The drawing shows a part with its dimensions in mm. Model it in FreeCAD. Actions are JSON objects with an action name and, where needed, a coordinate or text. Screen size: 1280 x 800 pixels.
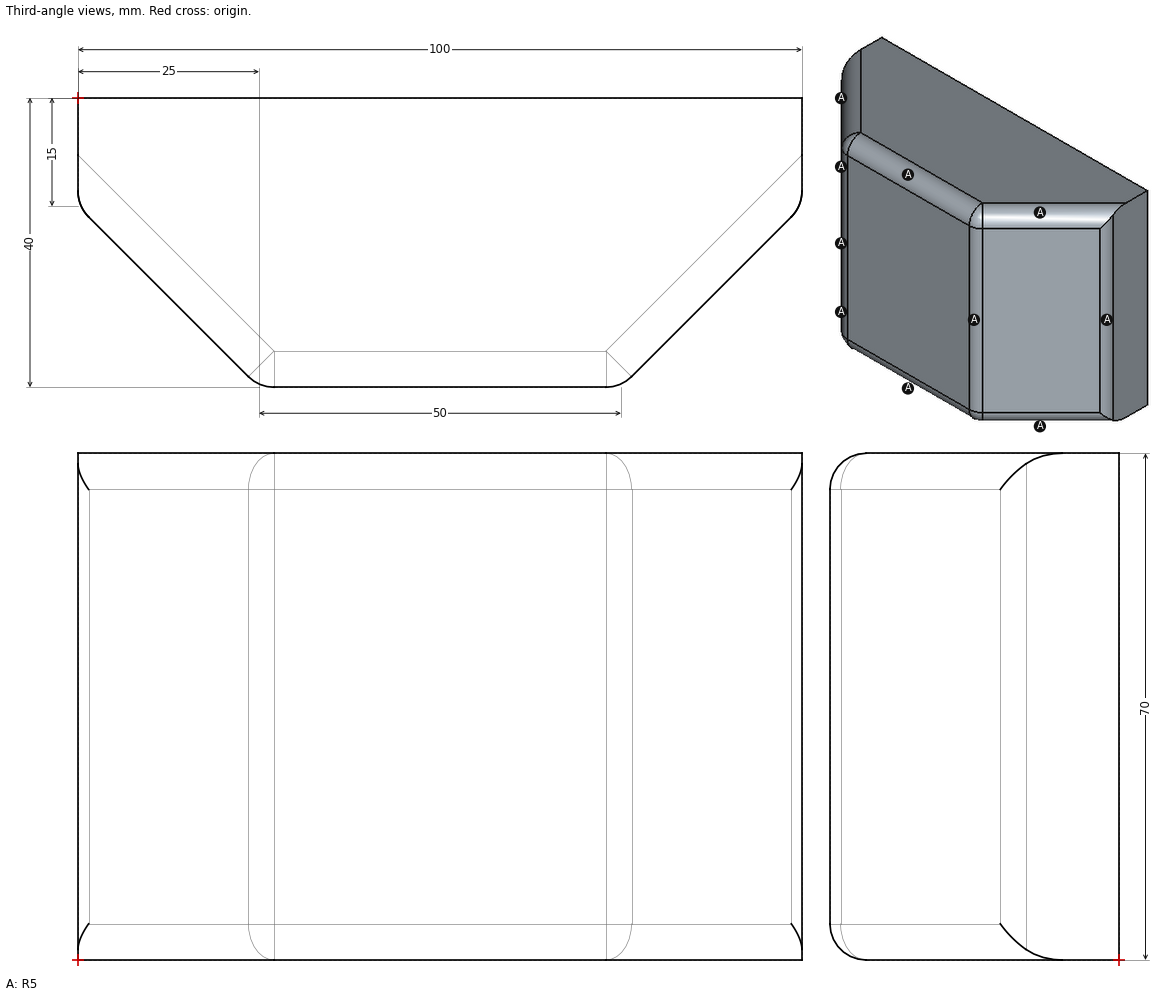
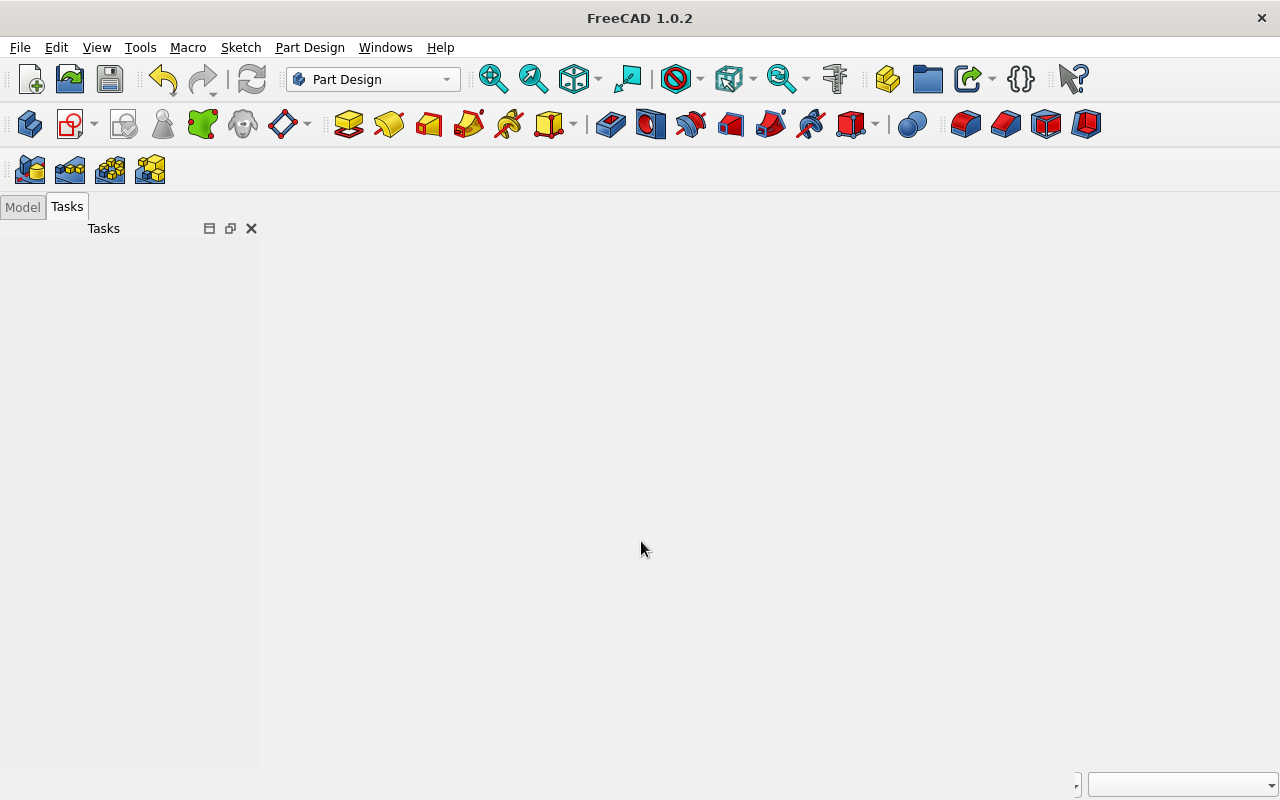
{"action": "key", "text": "ctrl+n"}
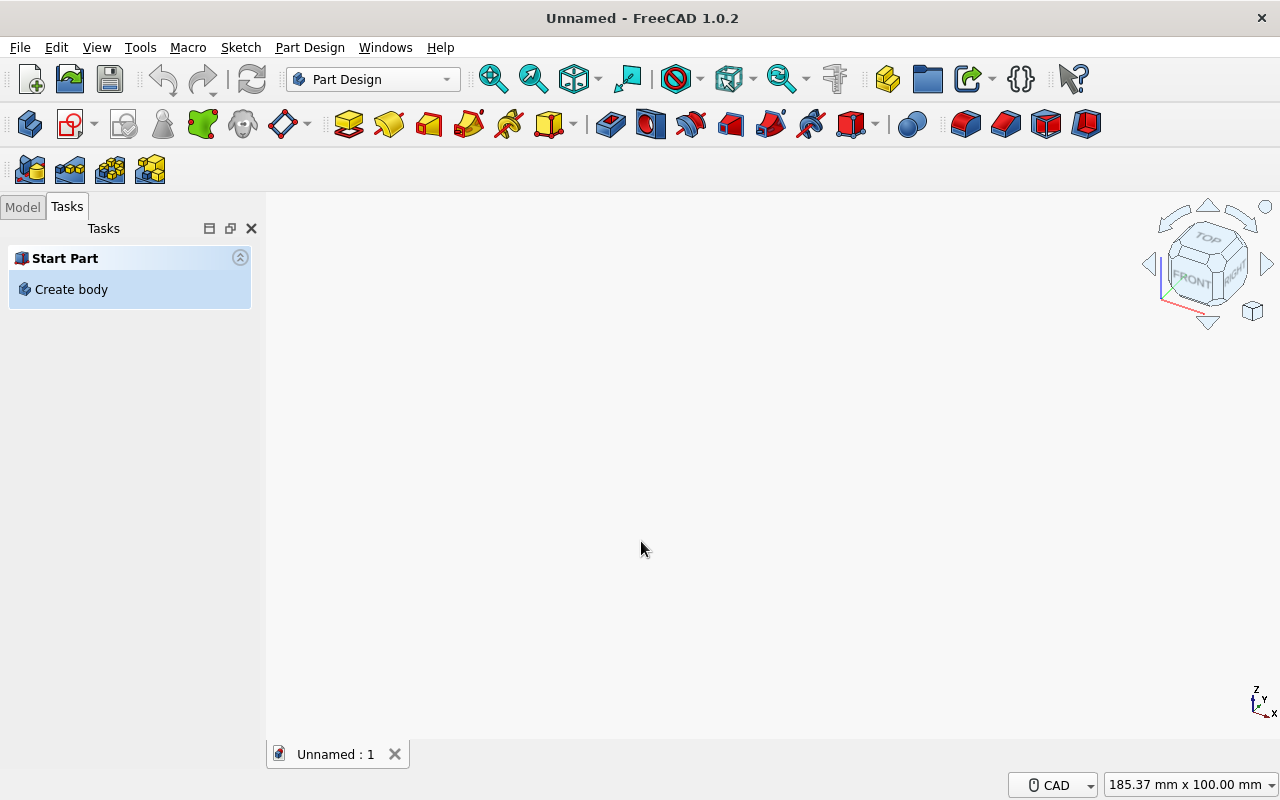
{"action": "left_click", "coordinate": [70, 124]}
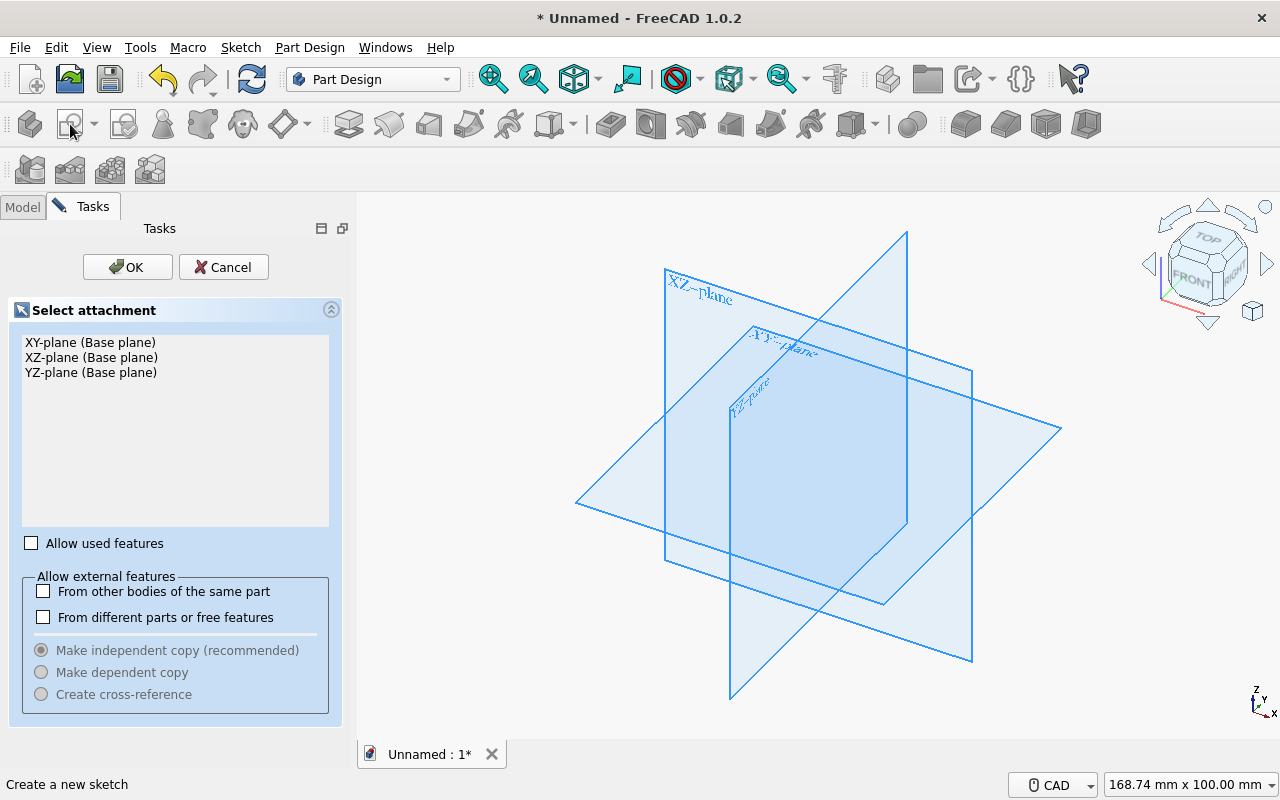
{"action": "left_click", "coordinate": [82, 342]}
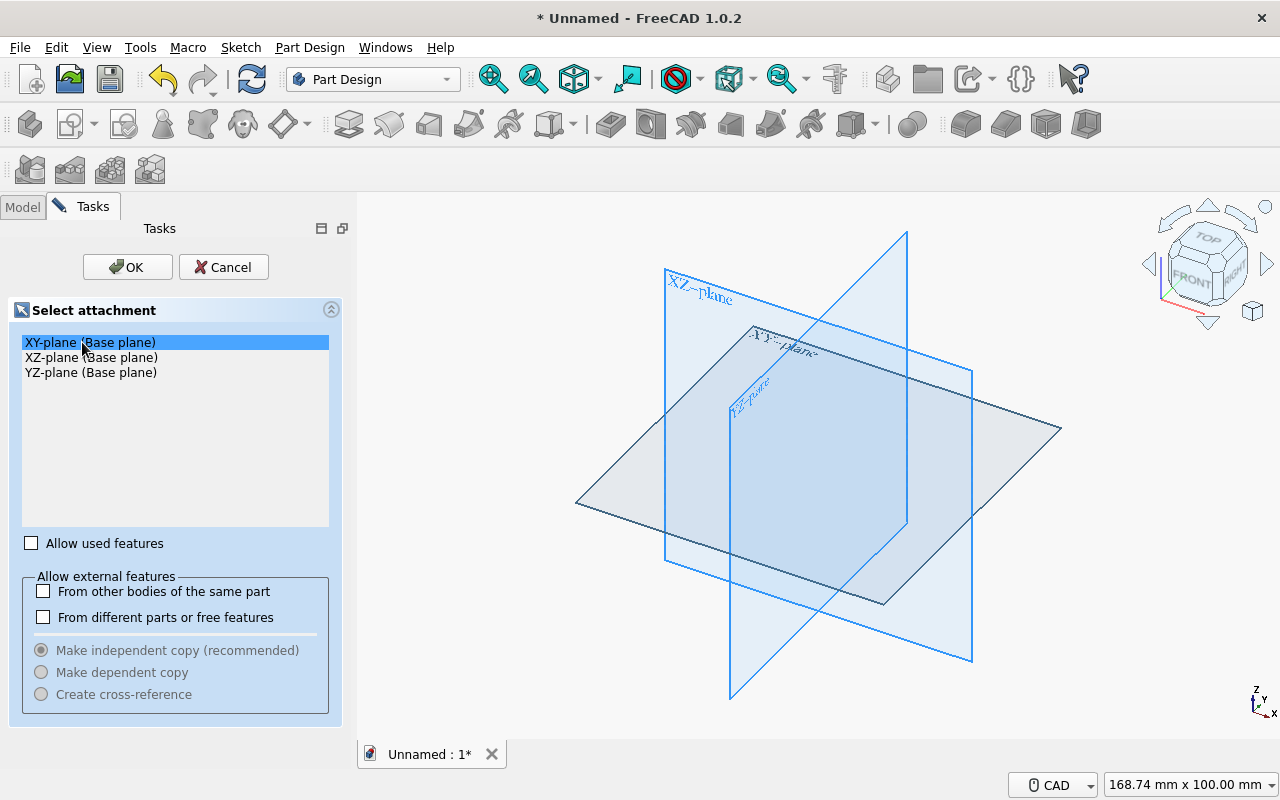
{"action": "left_click", "coordinate": [128, 267]}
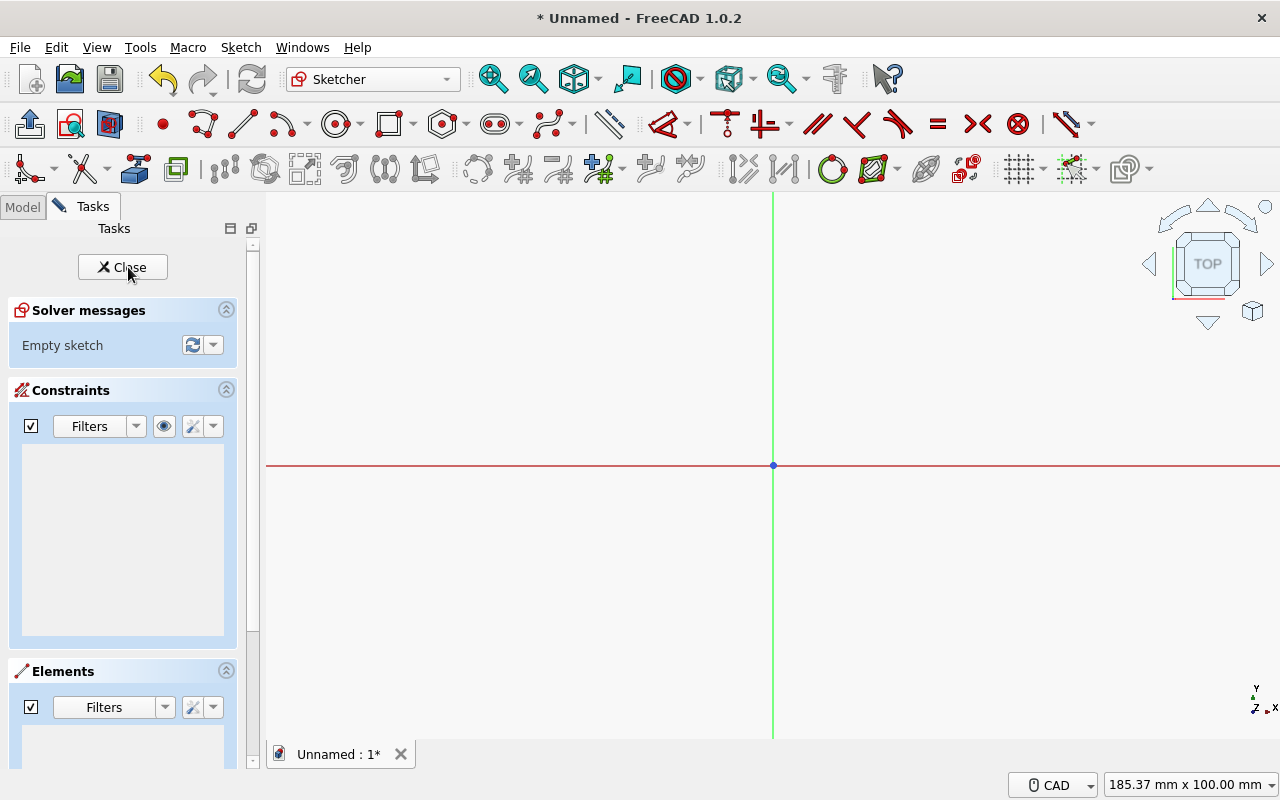
{"action": "scroll", "coordinate": [294, 243], "scroll_direction": "down", "scroll_amount": 2}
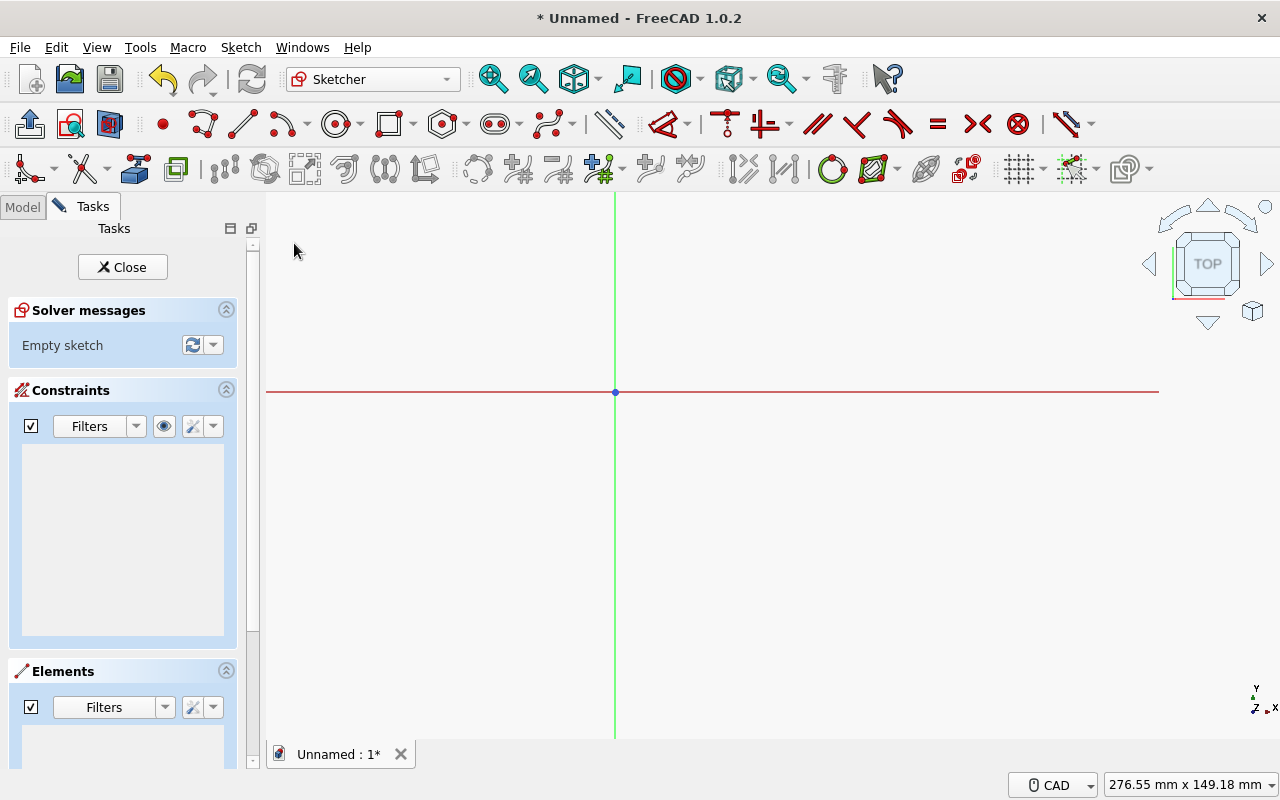
{"action": "scroll", "coordinate": [989, 466], "scroll_direction": "up", "scroll_amount": 2}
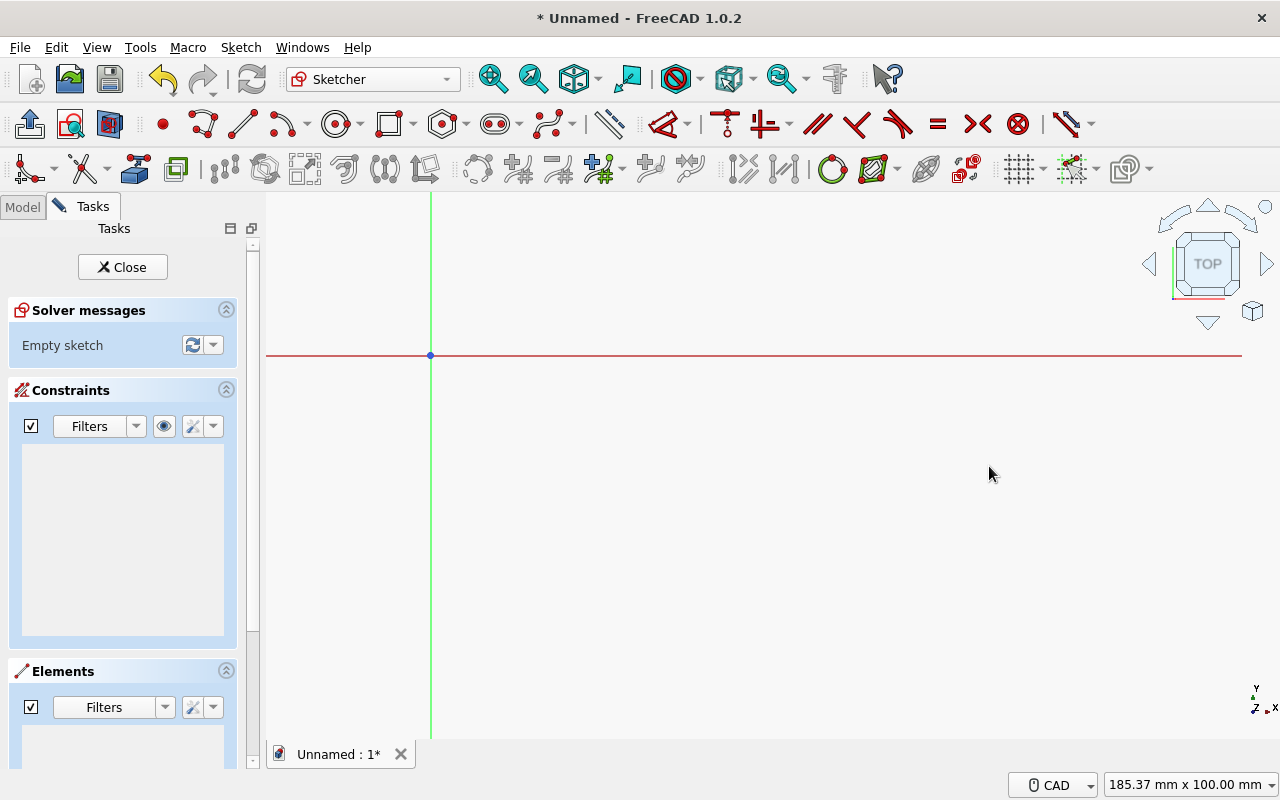
{"action": "left_click", "coordinate": [204, 124]}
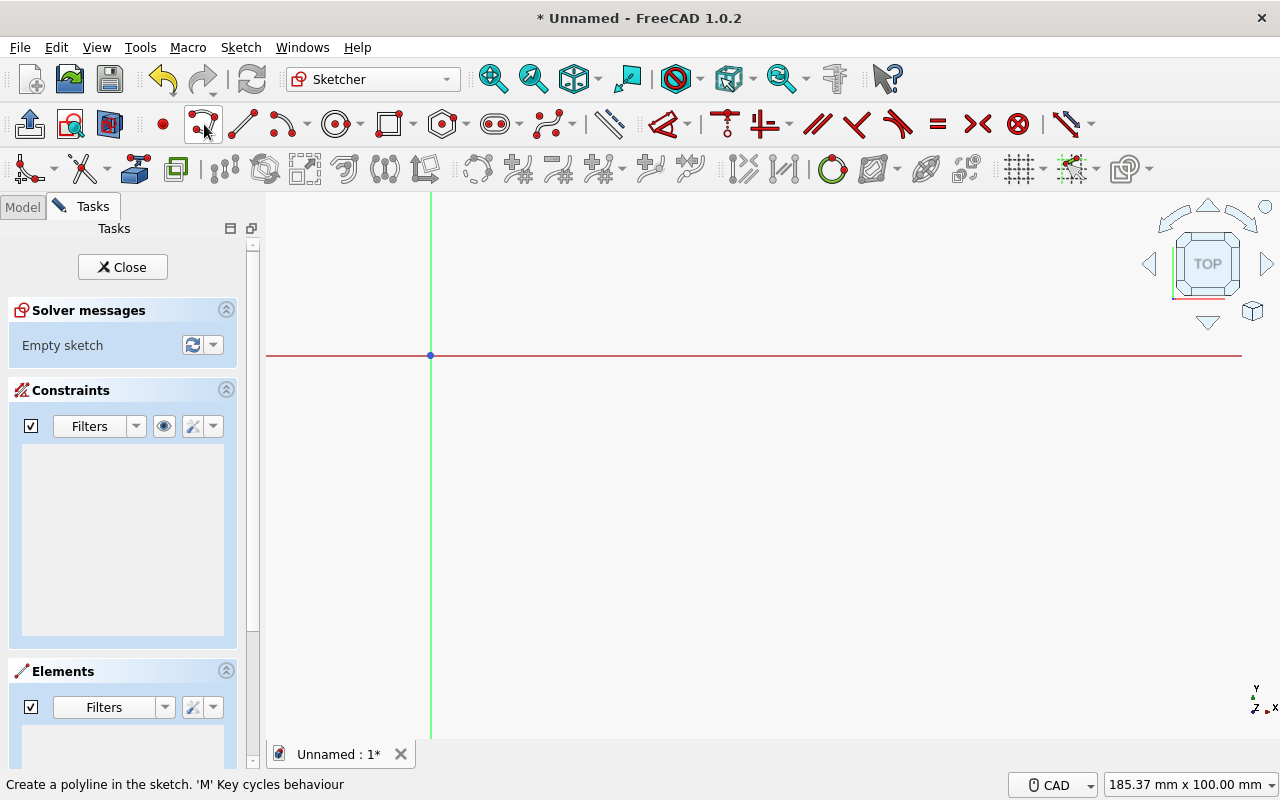
{"action": "left_click", "coordinate": [431, 356]}
{"action": "left_click", "coordinate": [440, 438]}
{"action": "left_click", "coordinate": [568, 574]}
{"action": "left_click", "coordinate": [841, 574]}
{"action": "left_click", "coordinate": [978, 438]}
{"action": "left_click", "coordinate": [978, 365]}
{"action": "left_click", "coordinate": [431, 356]}
{"action": "key", "text": "Escape"}
{"action": "key", "text": "Escape"}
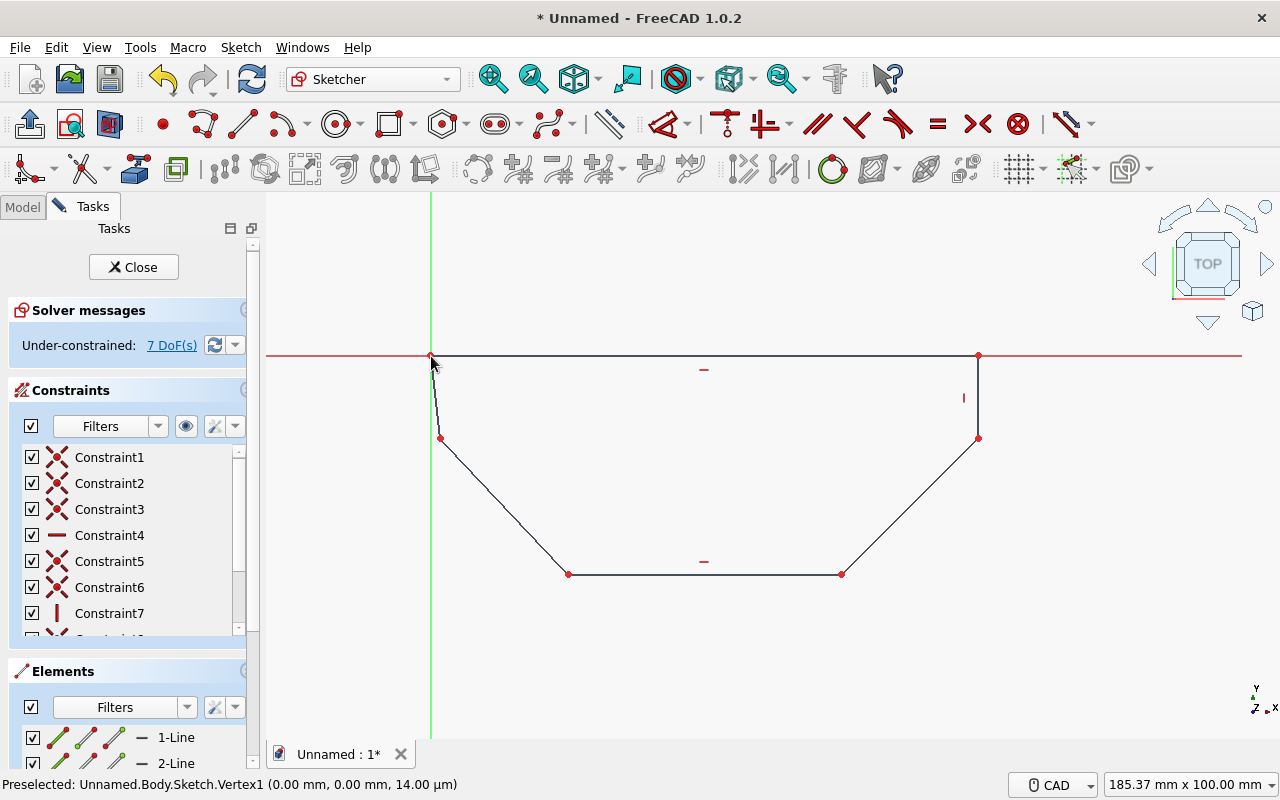
{"action": "left_click", "coordinate": [434, 381]}